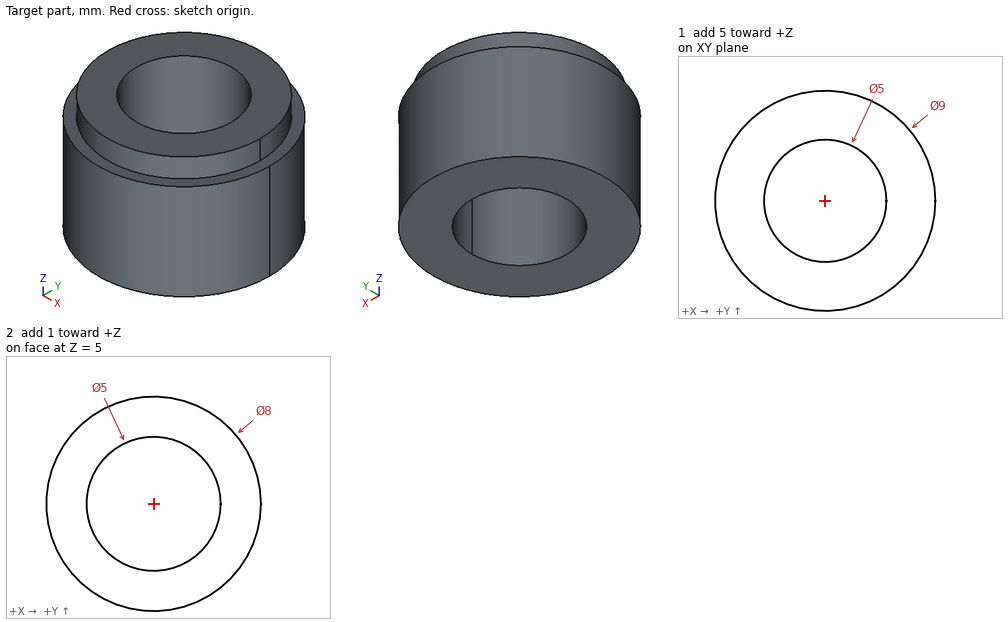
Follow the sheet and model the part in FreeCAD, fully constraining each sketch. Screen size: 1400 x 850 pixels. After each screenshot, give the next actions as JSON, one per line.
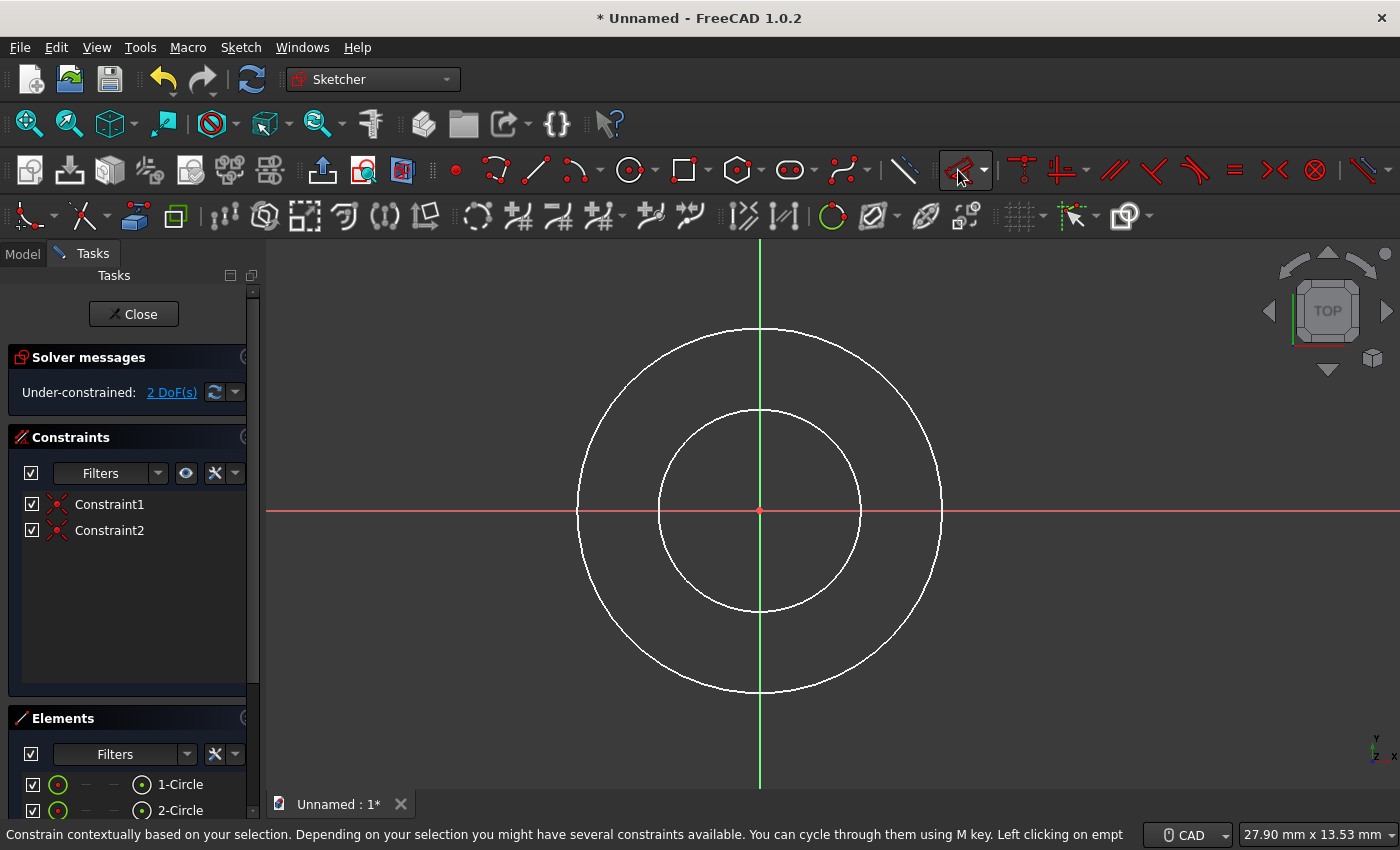
{"action": "left_click", "coordinate": [888, 381]}
{"action": "left_click", "coordinate": [910, 358]}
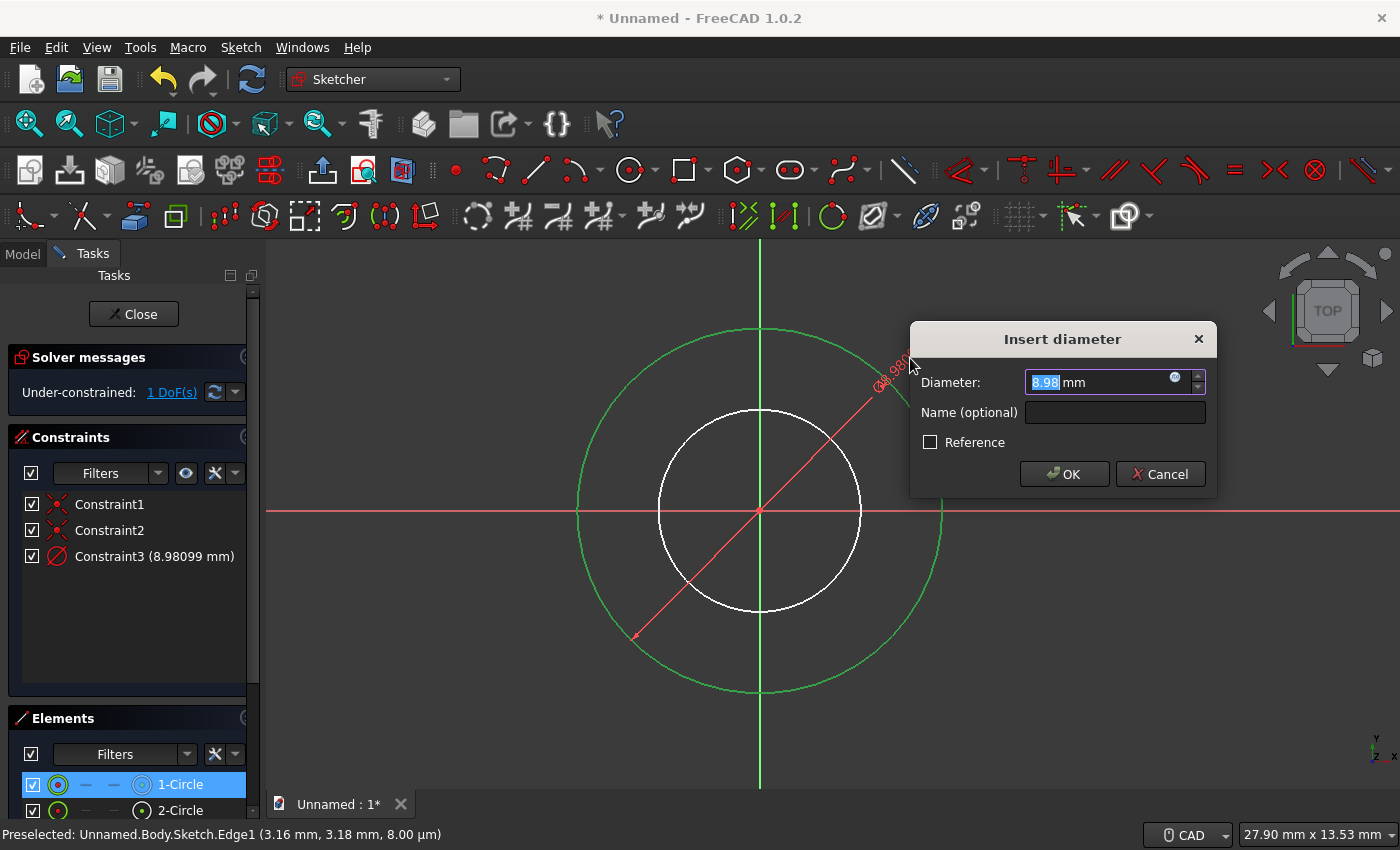
{"action": "type", "text": "9"}
{"action": "key", "text": "Return"}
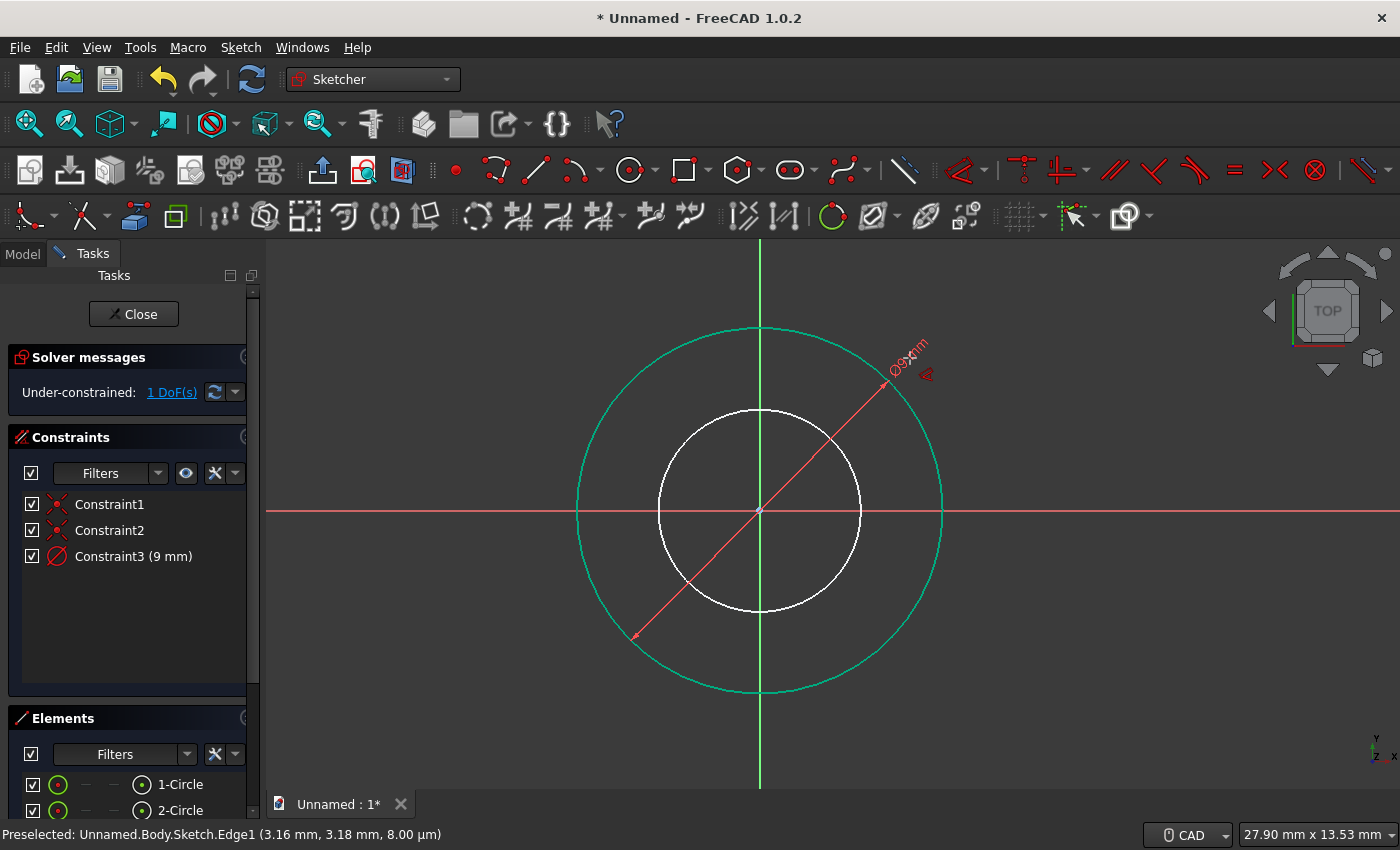
{"action": "left_click", "coordinate": [831, 439]}
{"action": "left_click", "coordinate": [854, 416]}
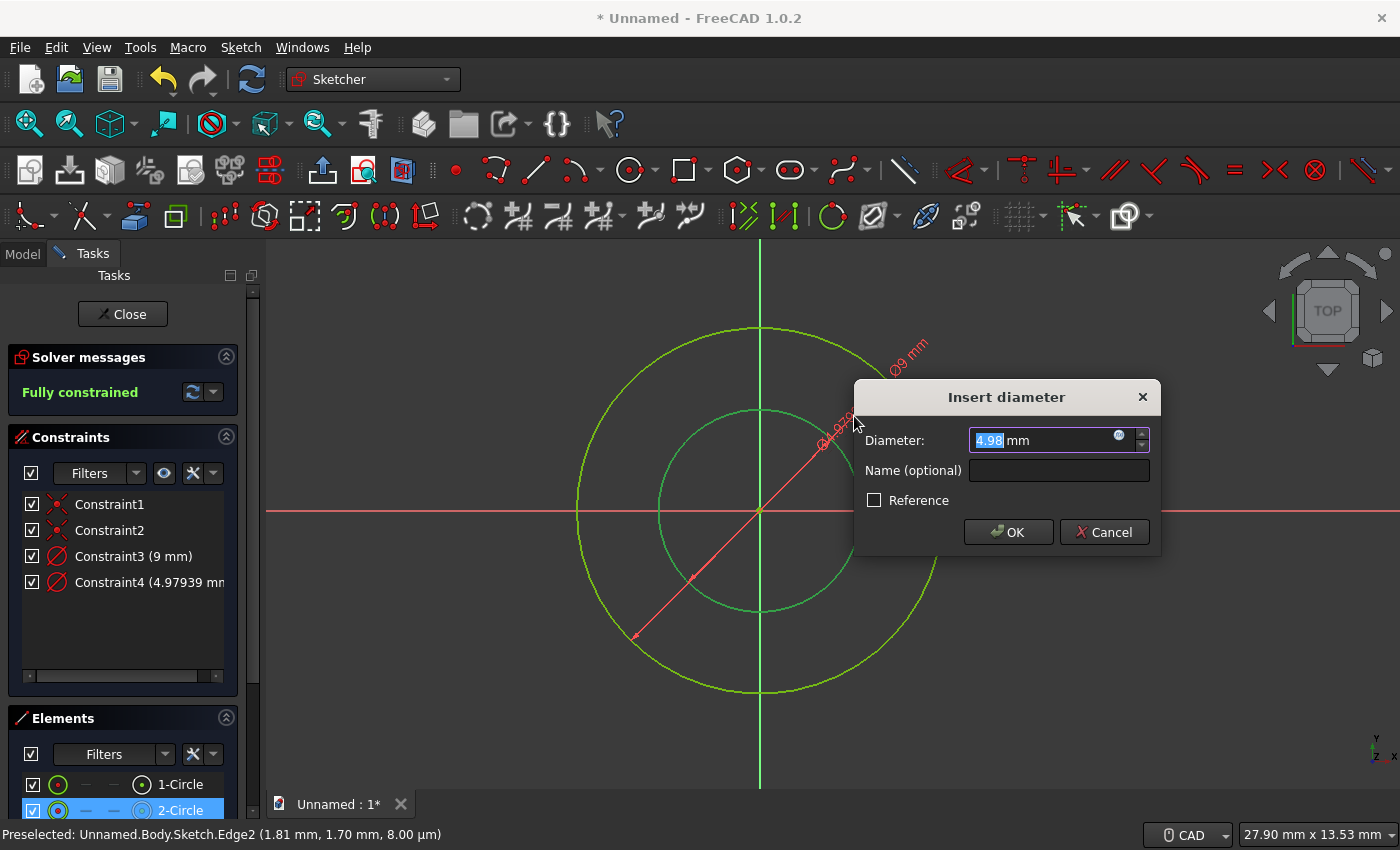
{"action": "type", "text": "5"}
{"action": "key", "text": "Return"}
{"action": "key", "text": "Escape"}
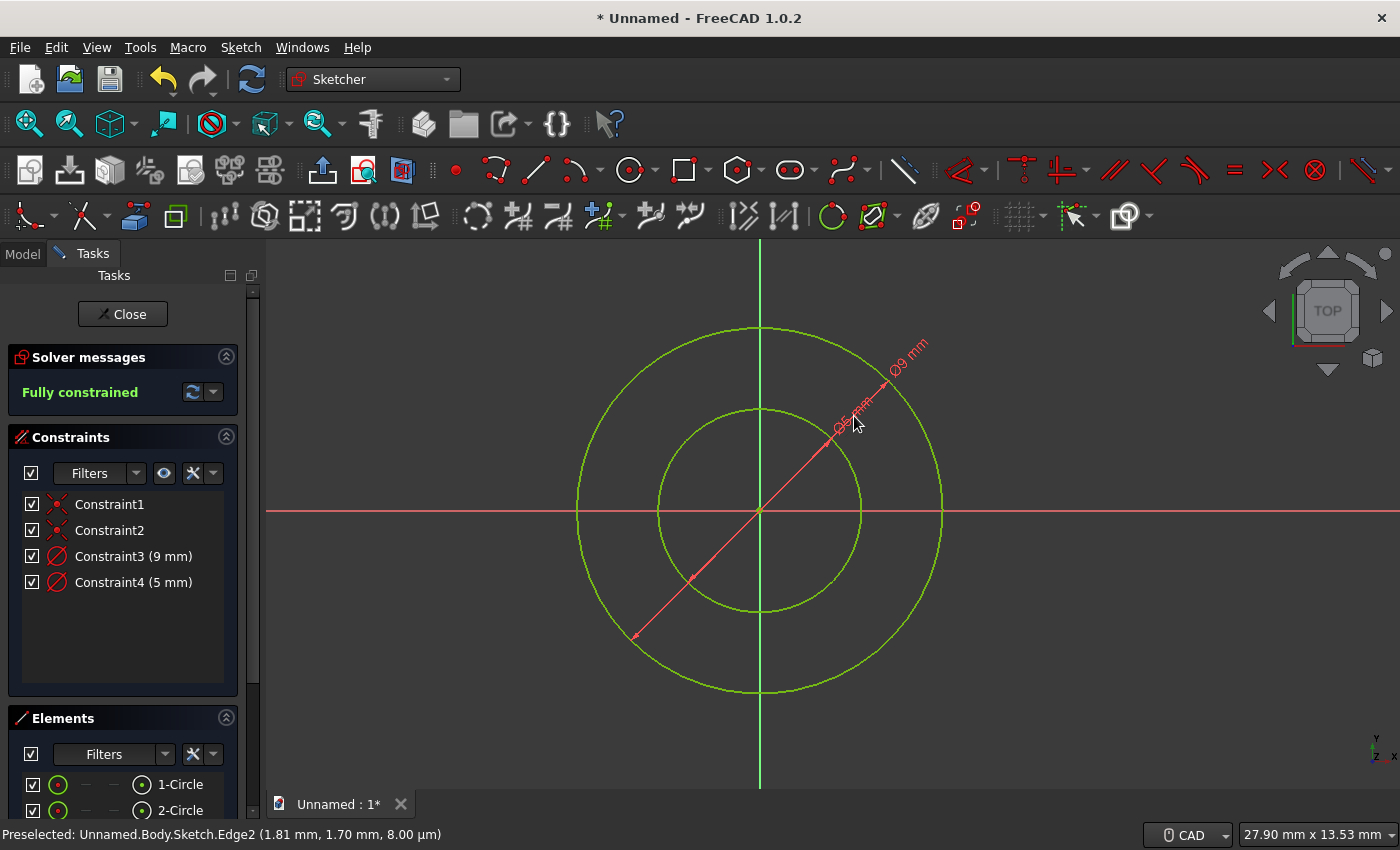
{"action": "left_click", "coordinate": [123, 314]}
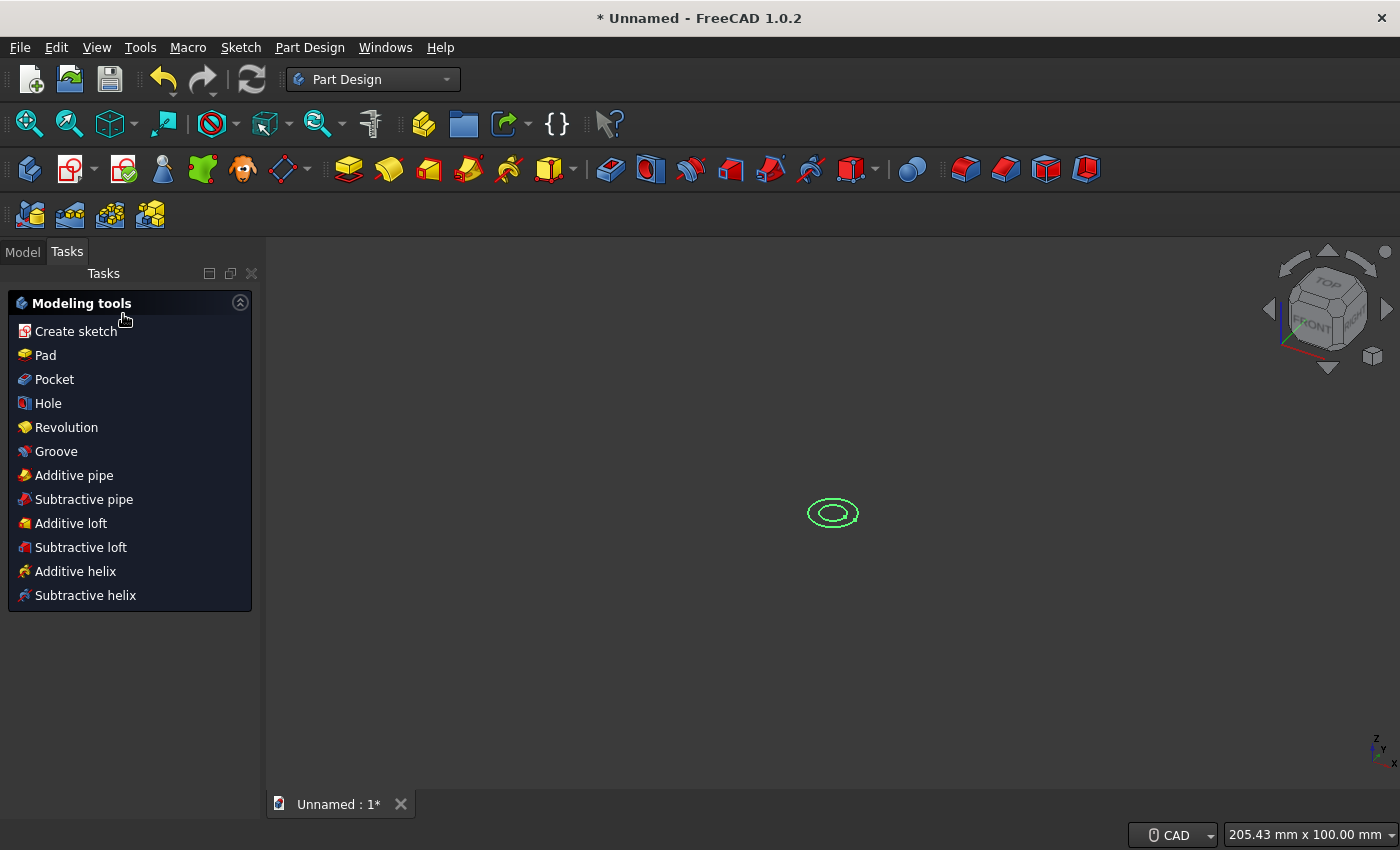
{"action": "left_click", "coordinate": [350, 170]}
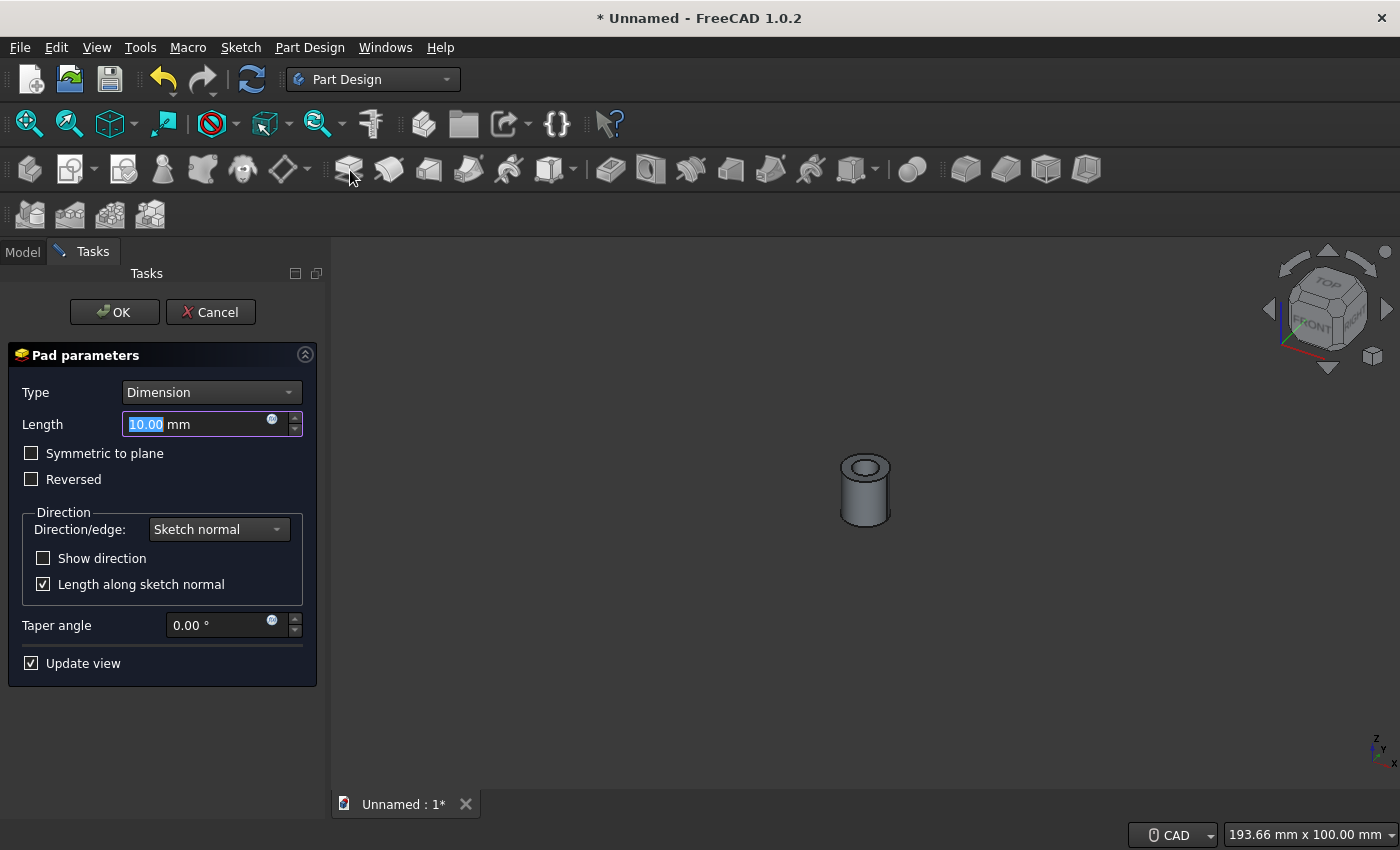
{"action": "type", "text": "5"}
{"action": "key", "text": "Tab"}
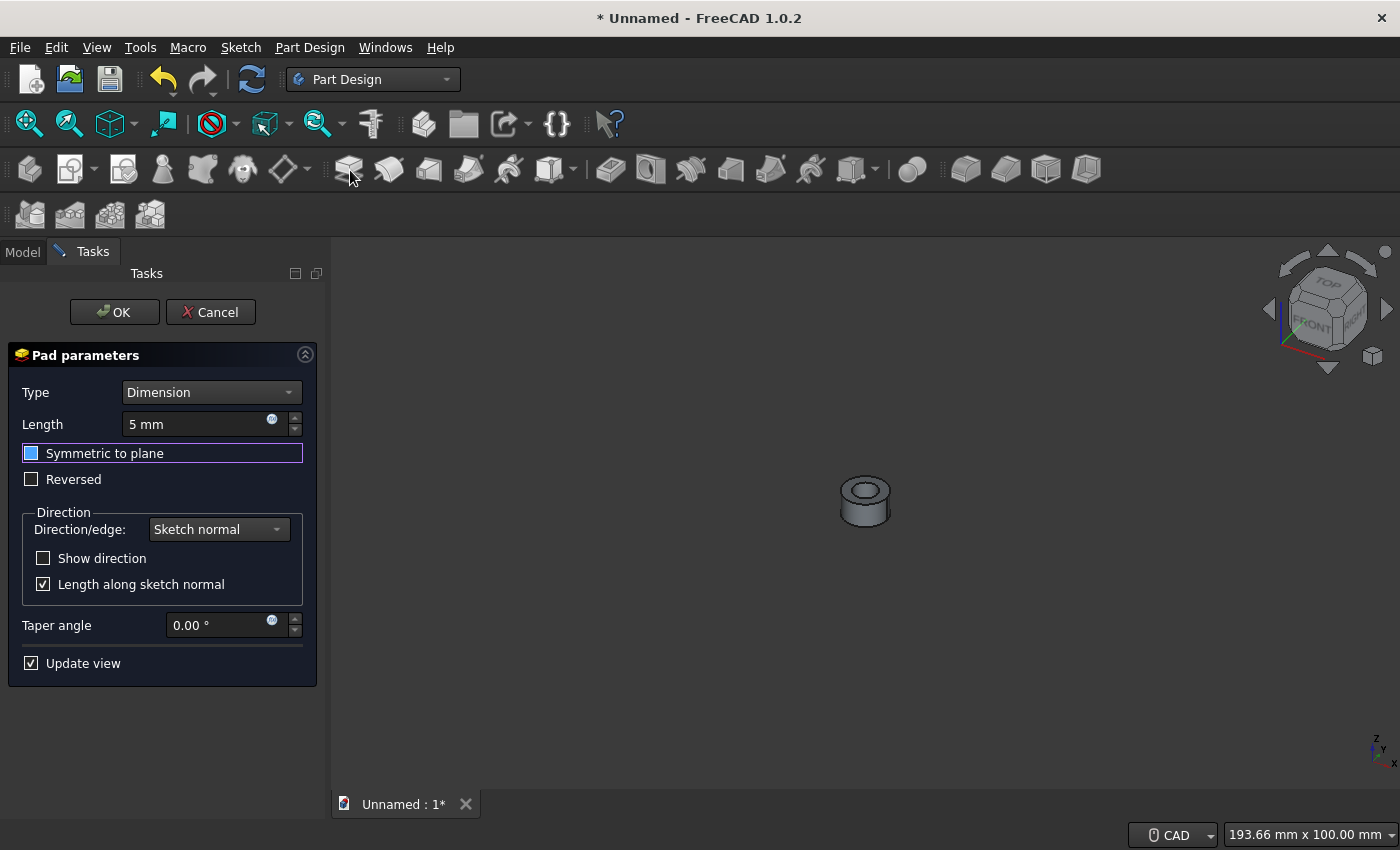
{"action": "left_click", "coordinate": [115, 312]}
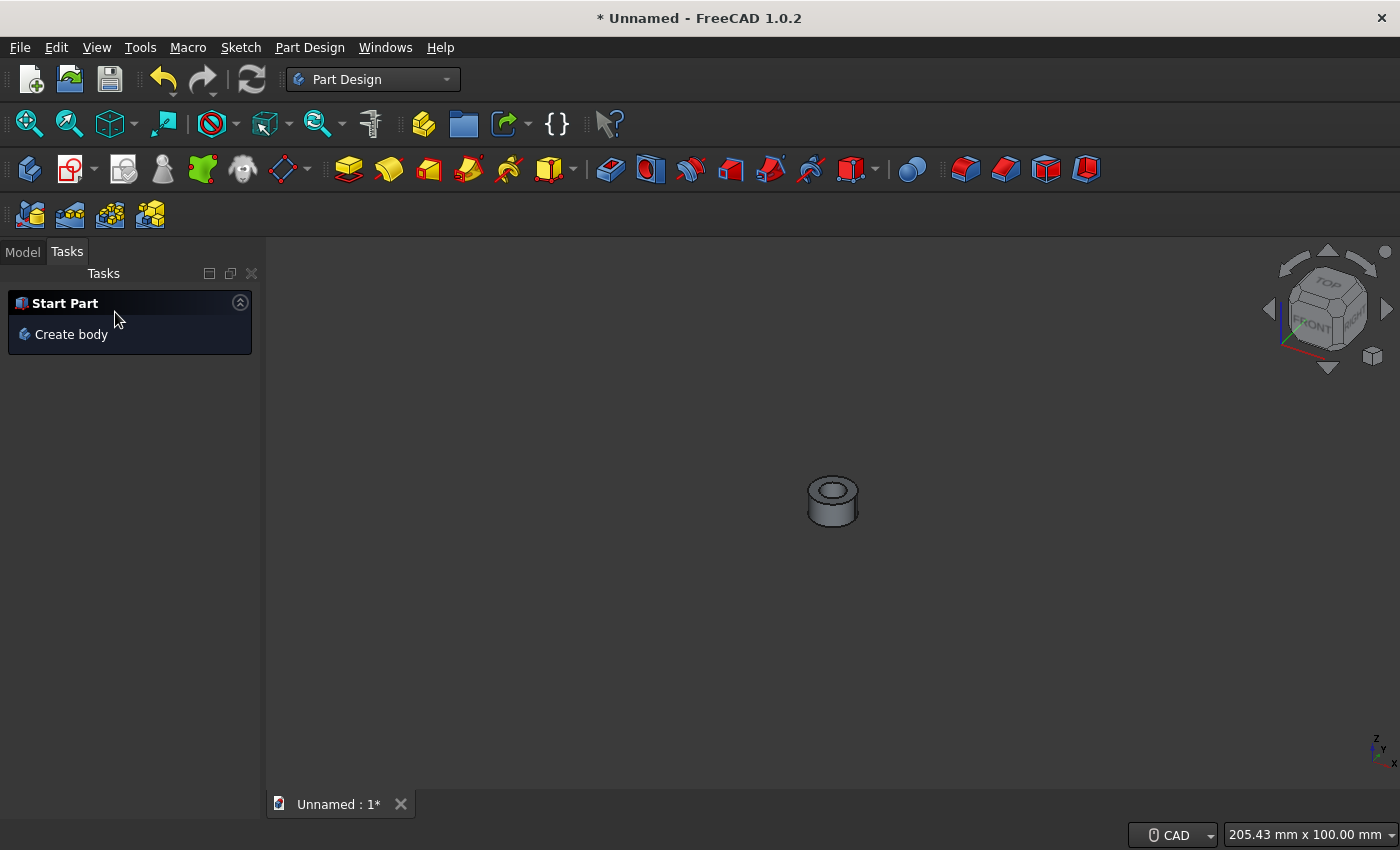
{"action": "left_click", "coordinate": [30, 124]}